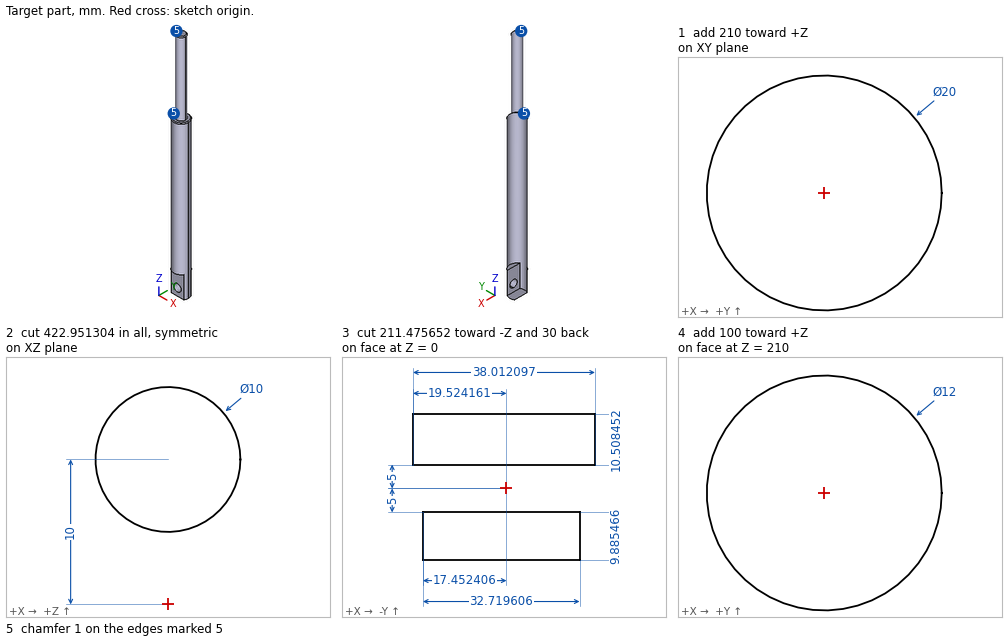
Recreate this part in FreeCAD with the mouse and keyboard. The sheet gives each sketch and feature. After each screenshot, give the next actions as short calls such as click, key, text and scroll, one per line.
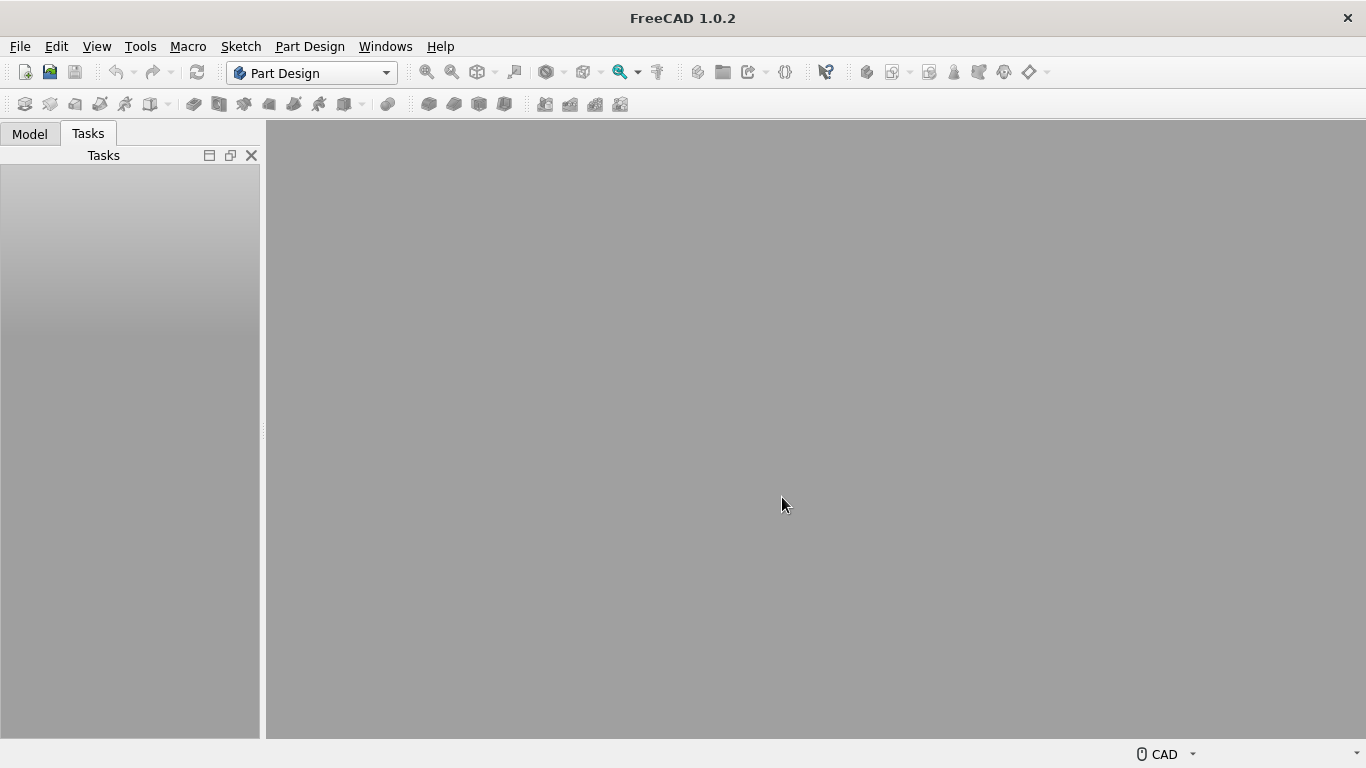
click(25, 72)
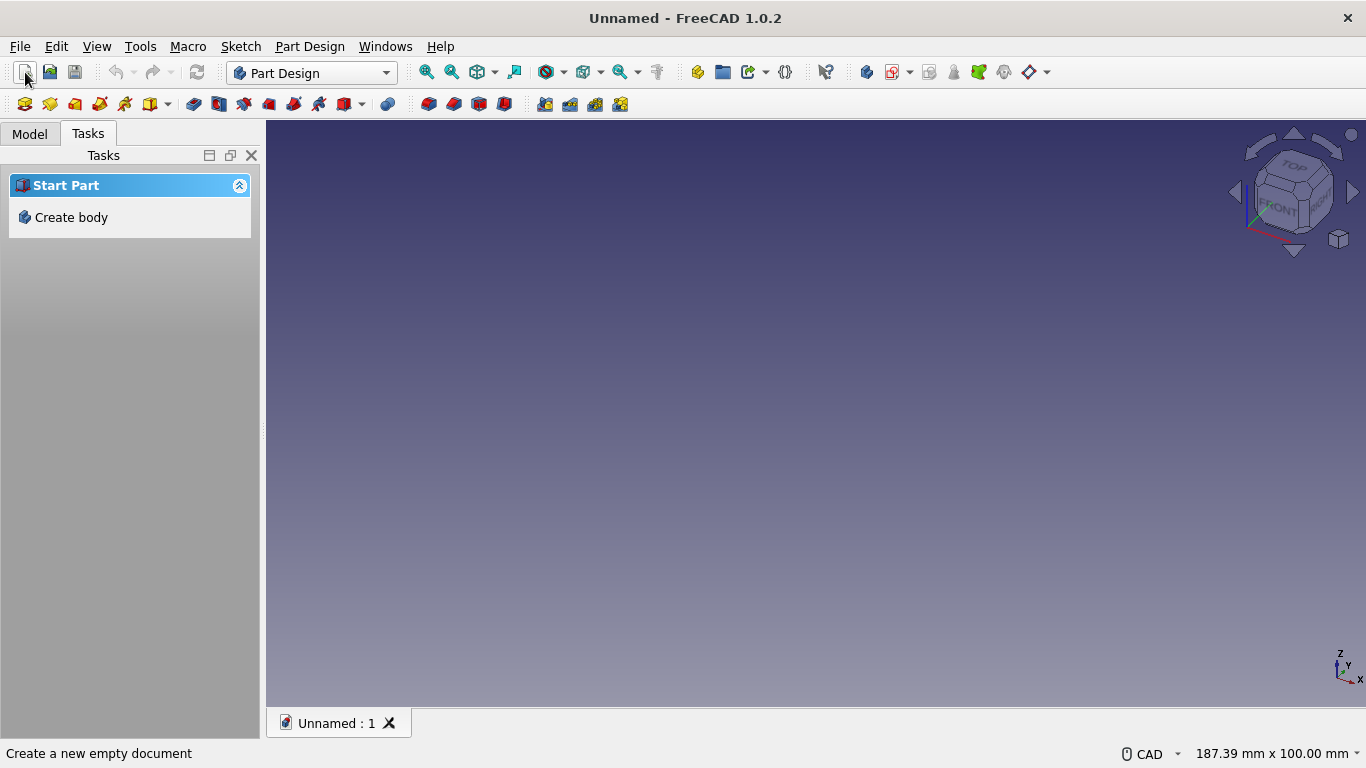
click(892, 72)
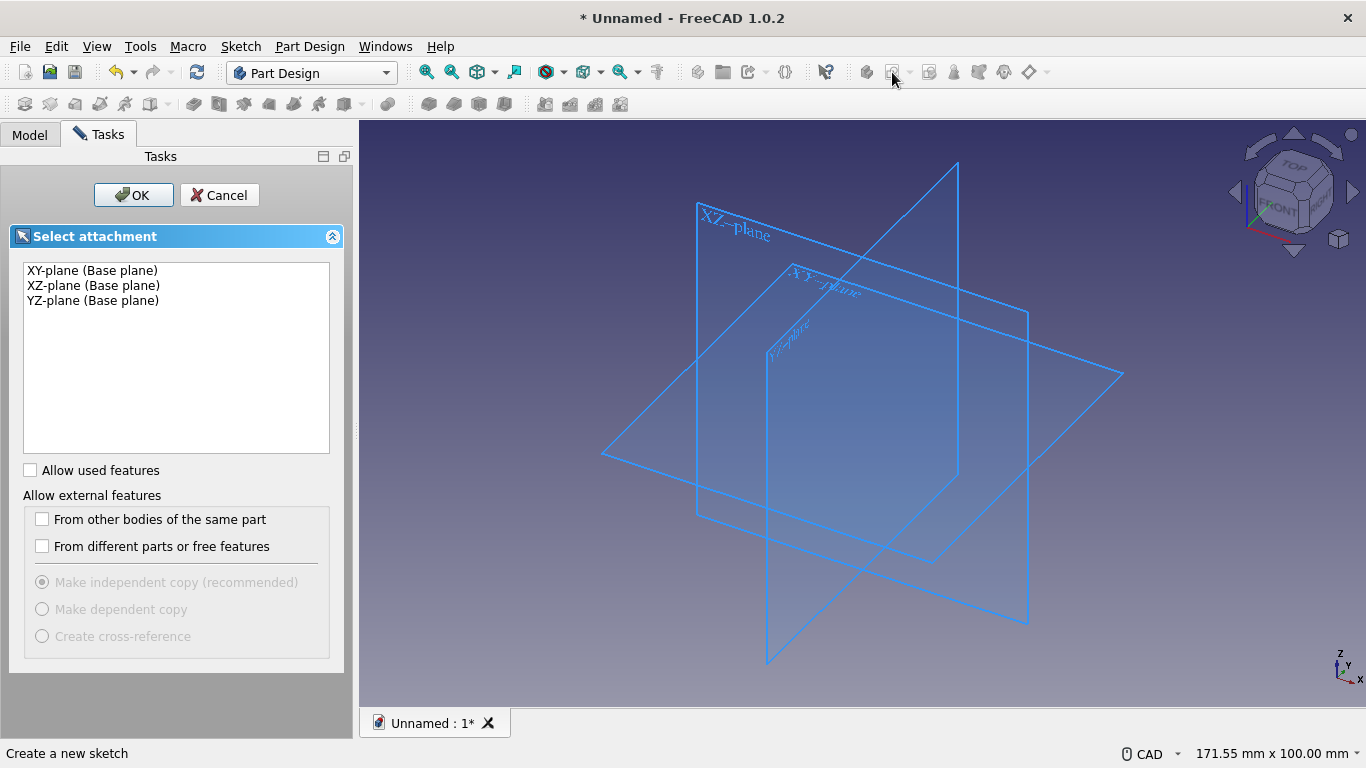
click(84, 270)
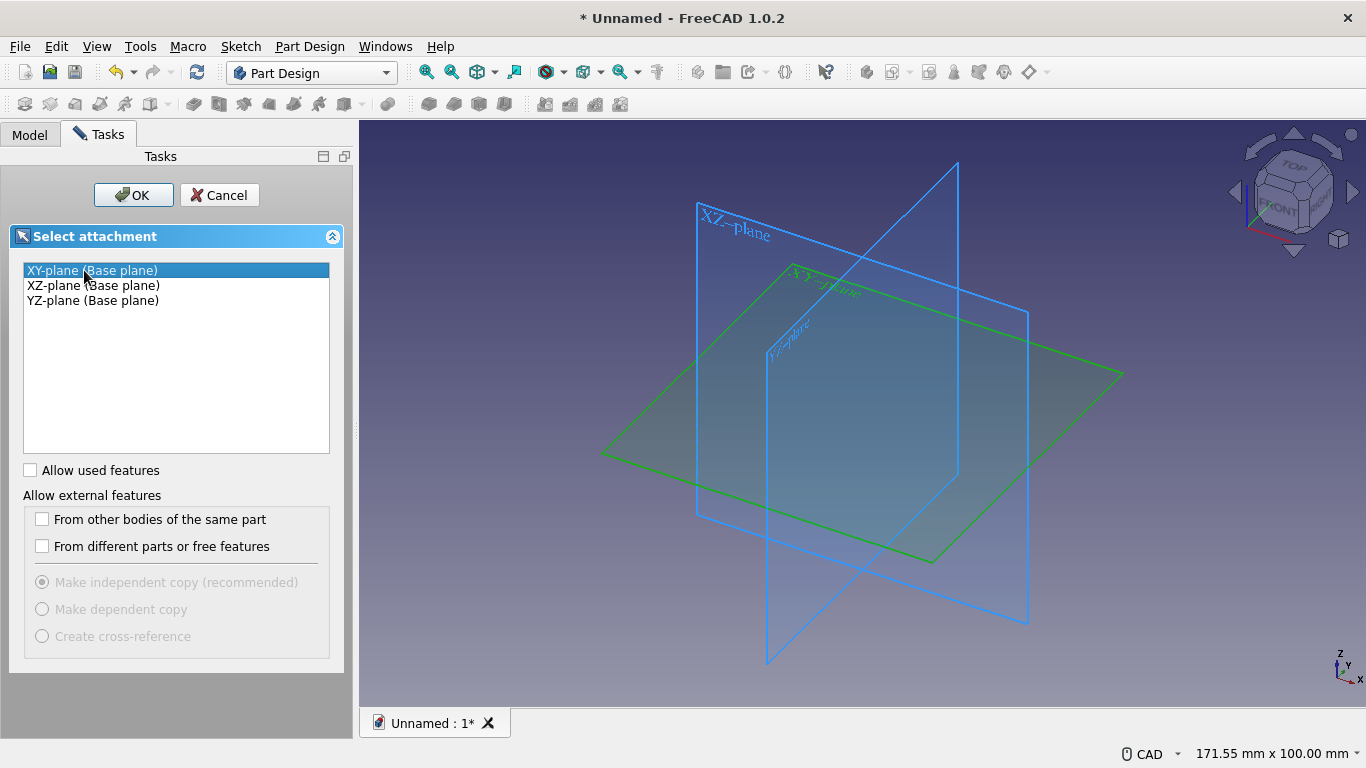
click(134, 195)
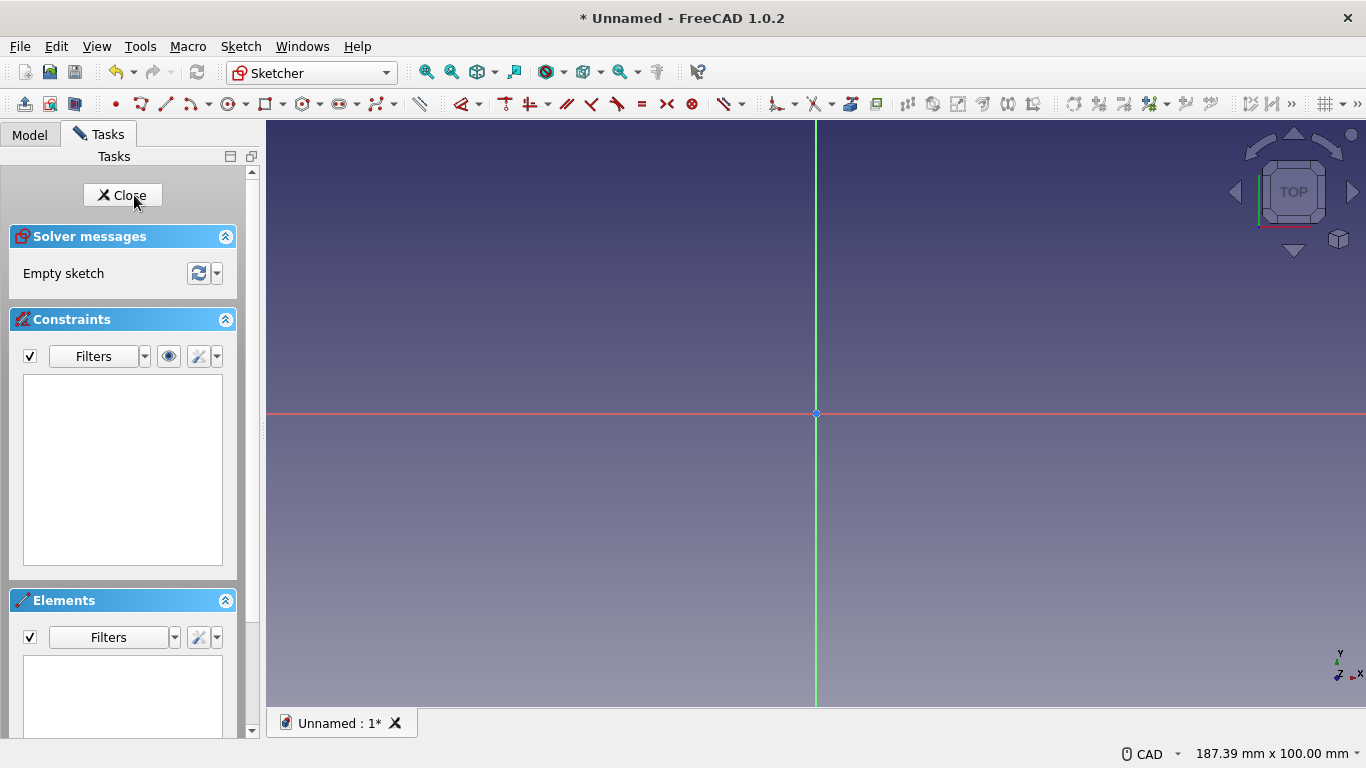
scroll(846, 414, up, 6)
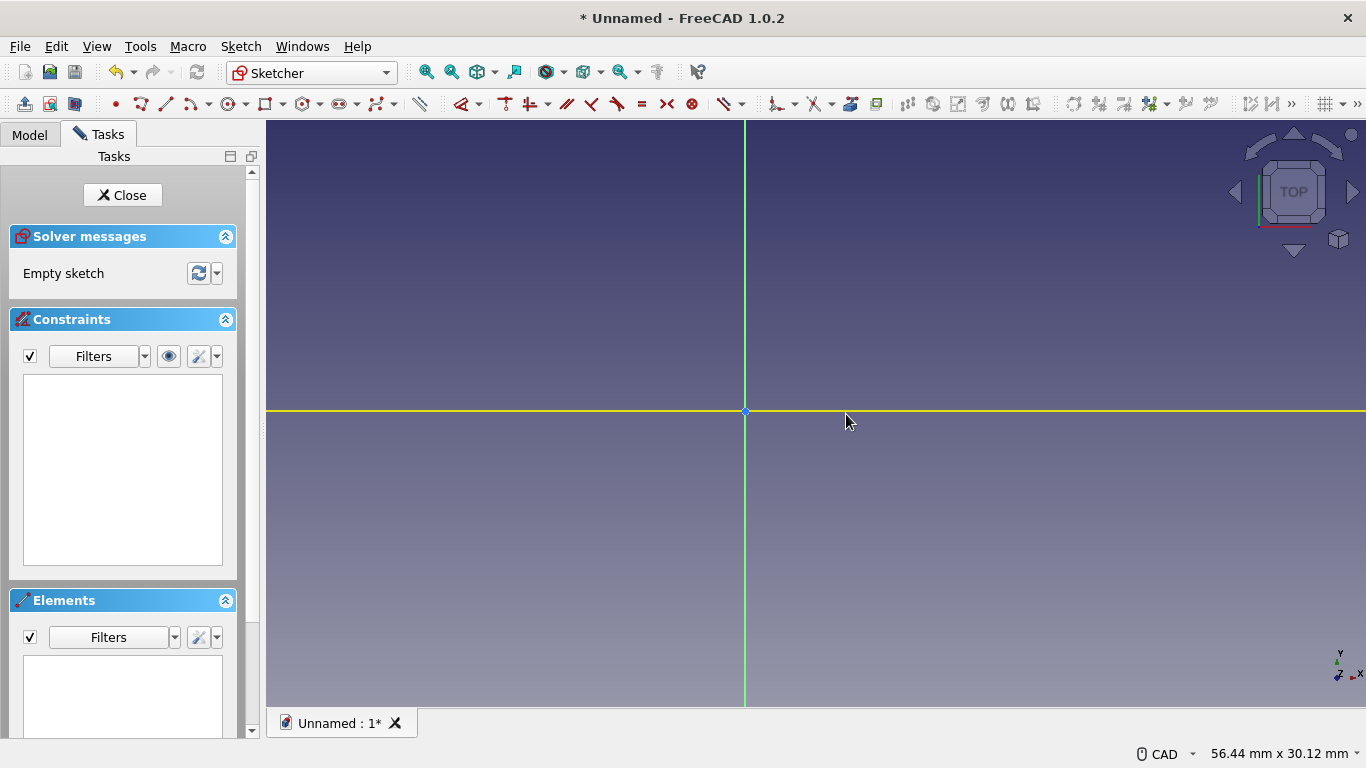
click(228, 104)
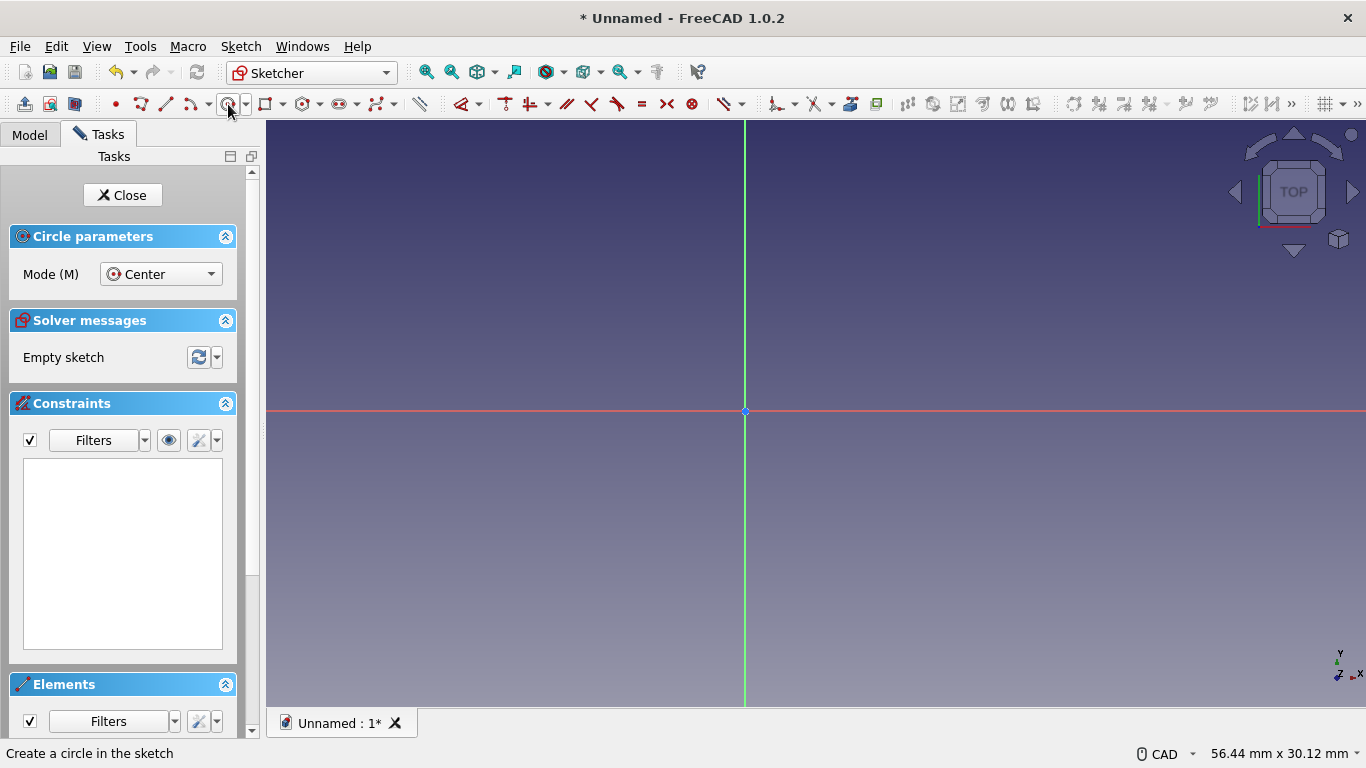
click(745, 411)
move(883, 273)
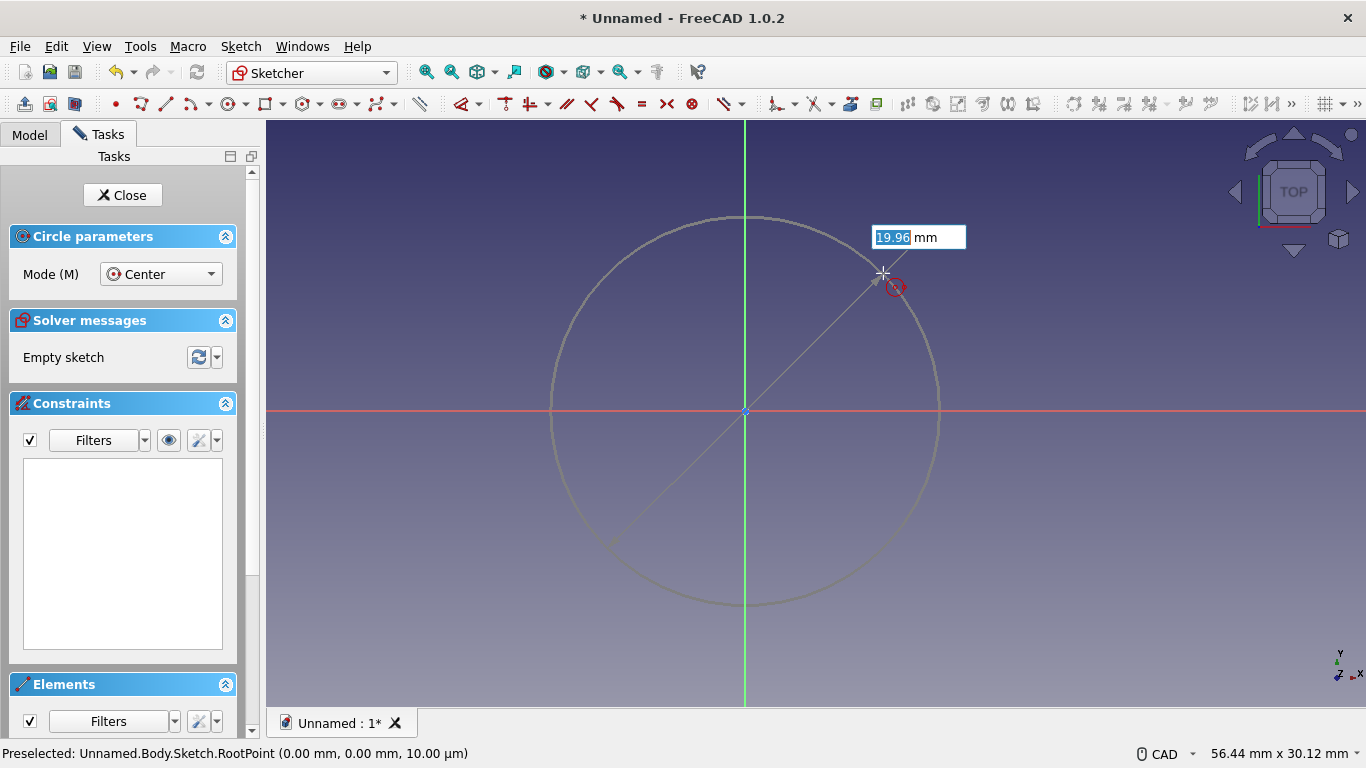
text(20)
key(Return)
key(Escape)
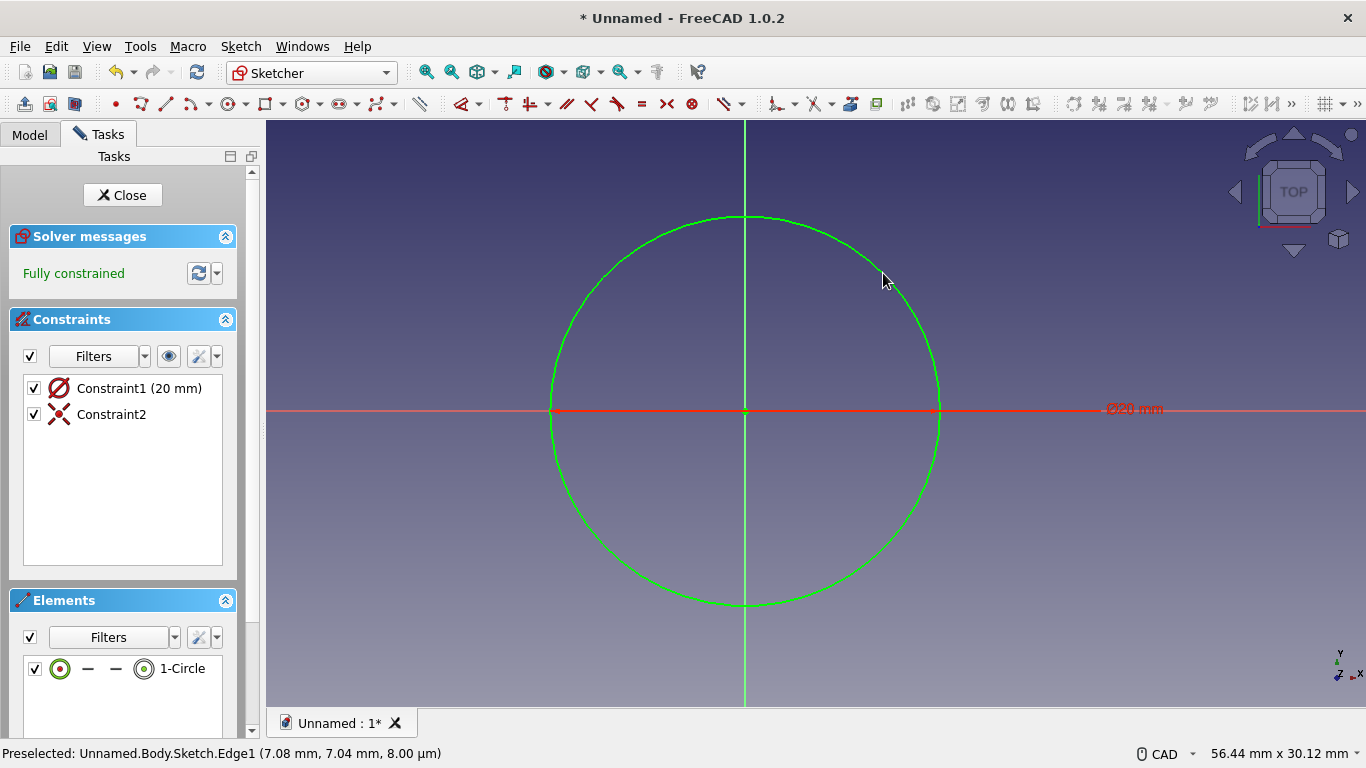
click(123, 195)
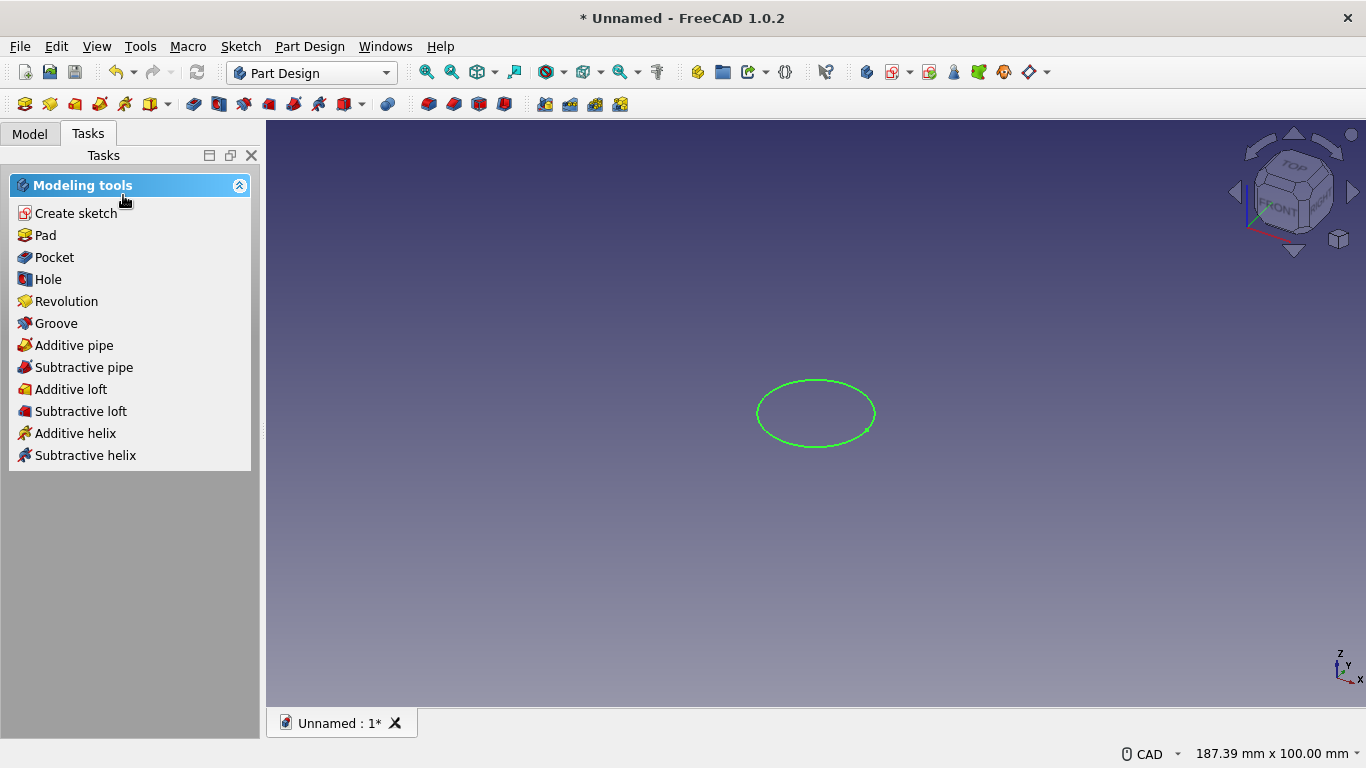
click(25, 104)